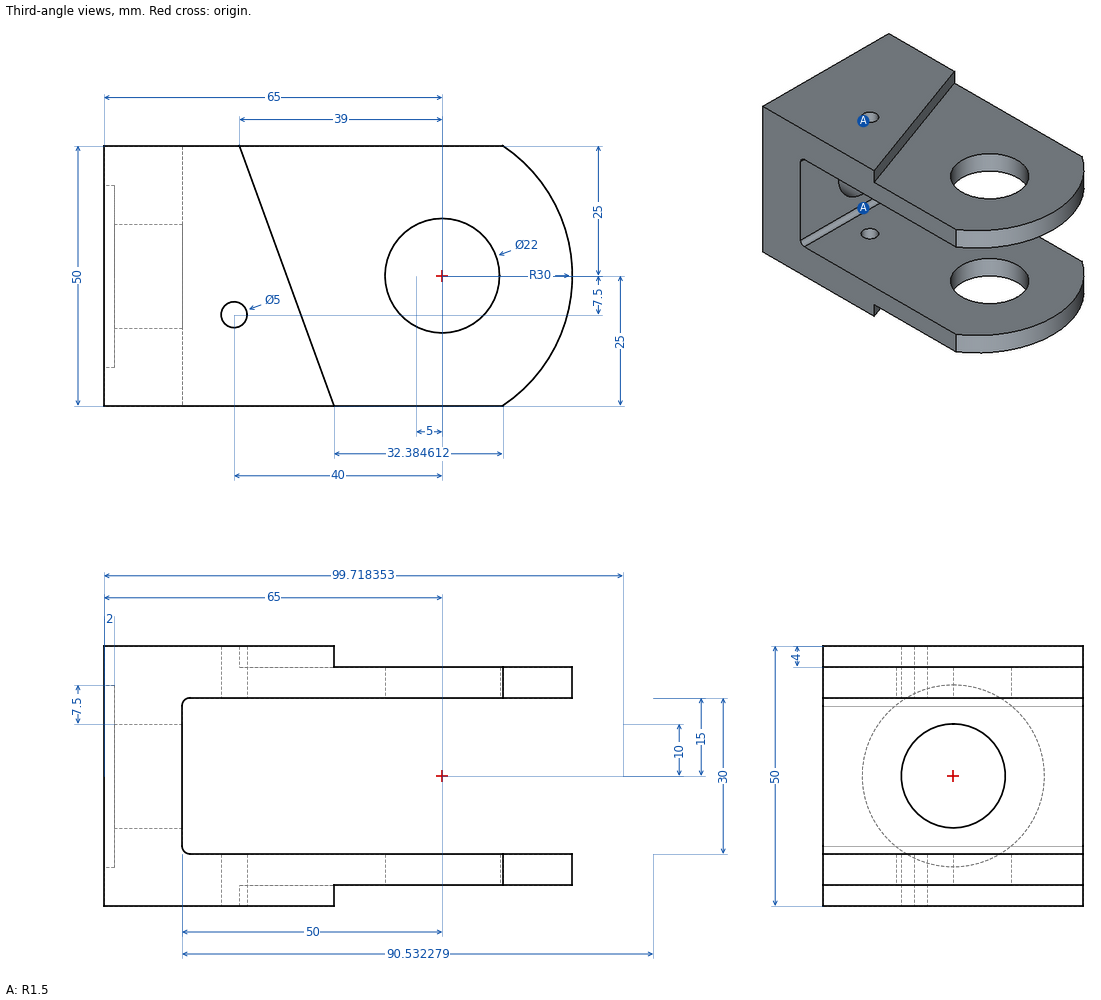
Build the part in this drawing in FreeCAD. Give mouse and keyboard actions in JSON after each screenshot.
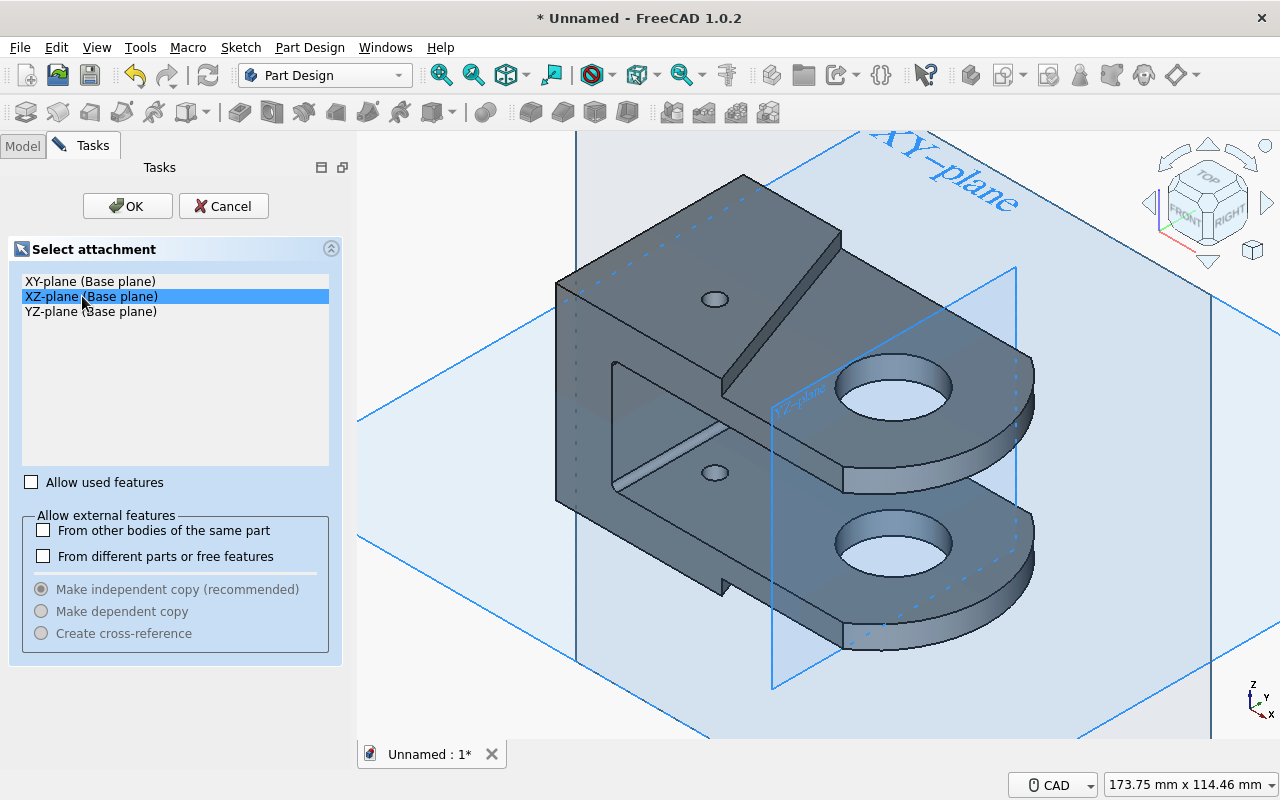
{"action": "left_click", "coordinate": [128, 206]}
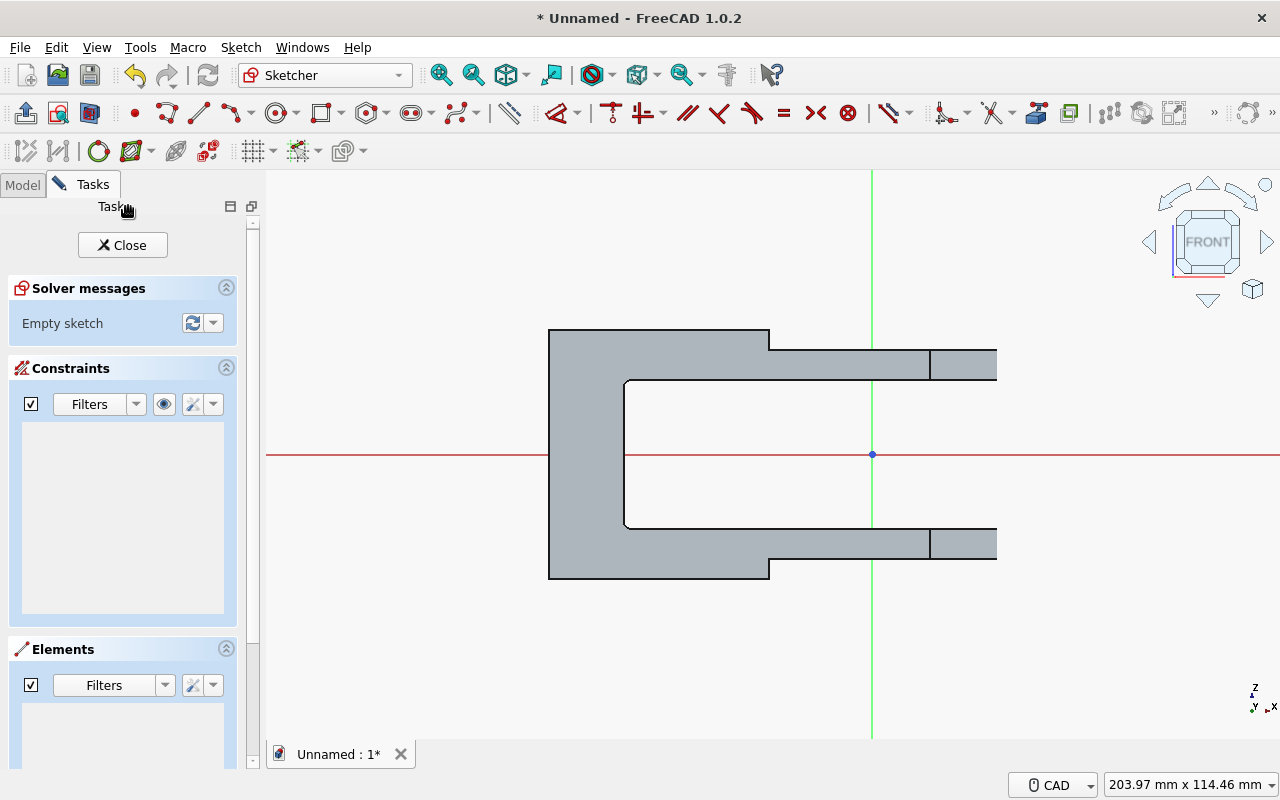
{"action": "left_click", "coordinate": [90, 114]}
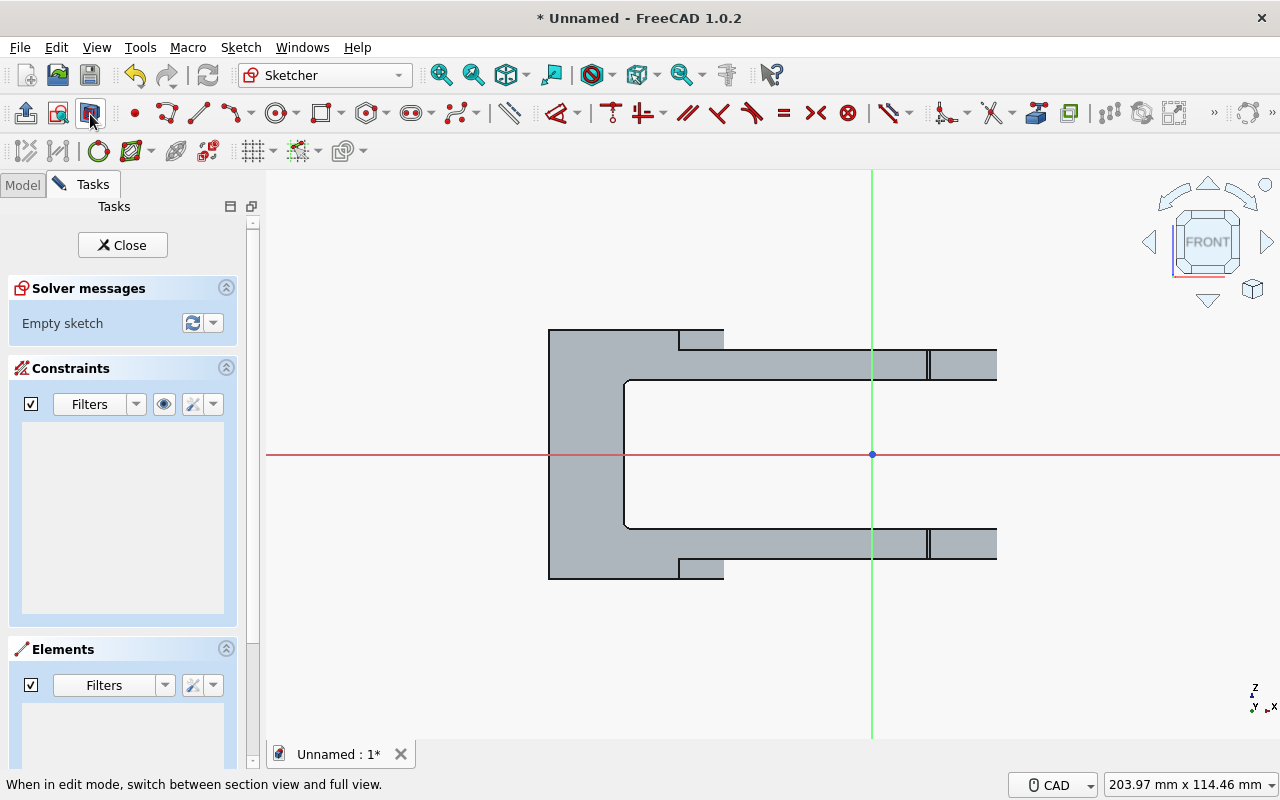
{"action": "left_click", "coordinate": [168, 114]}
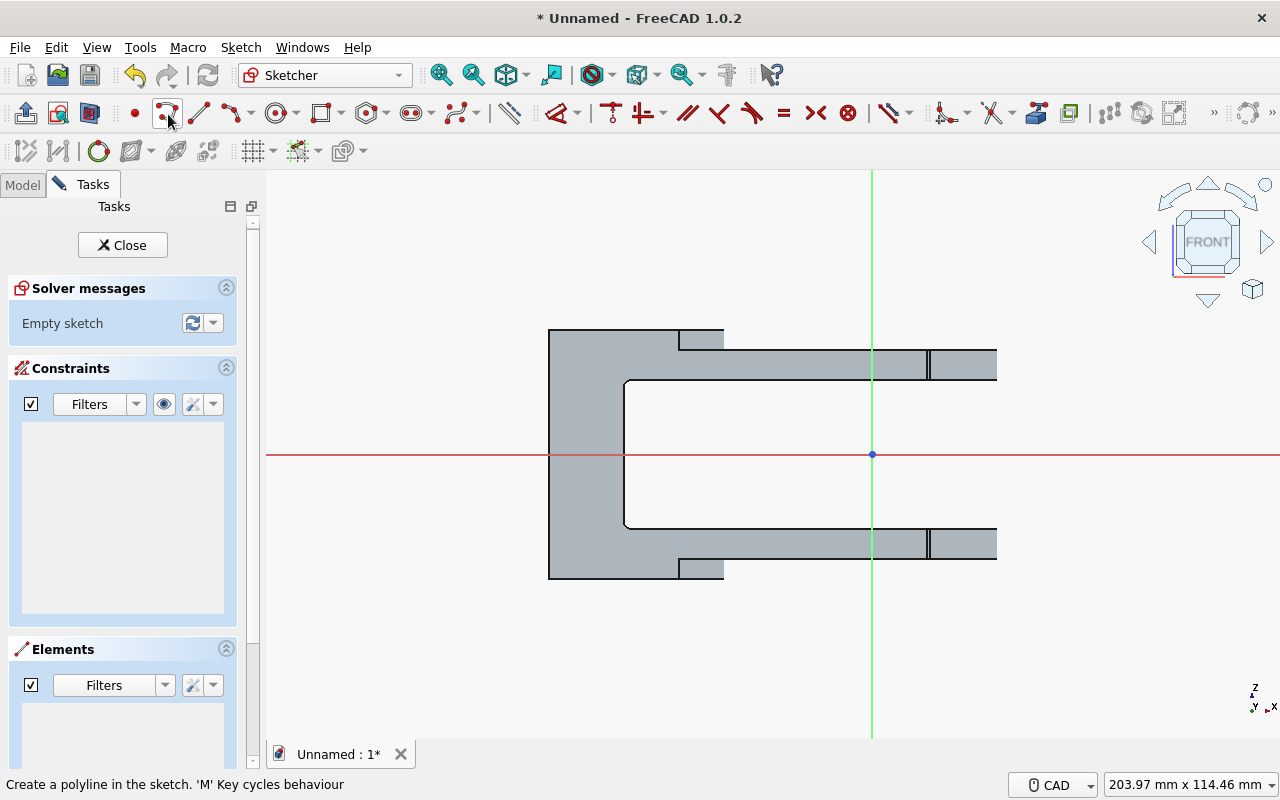
{"action": "left_click", "coordinate": [1045, 454]}
{"action": "left_click", "coordinate": [549, 446]}
{"action": "left_click", "coordinate": [549, 368]}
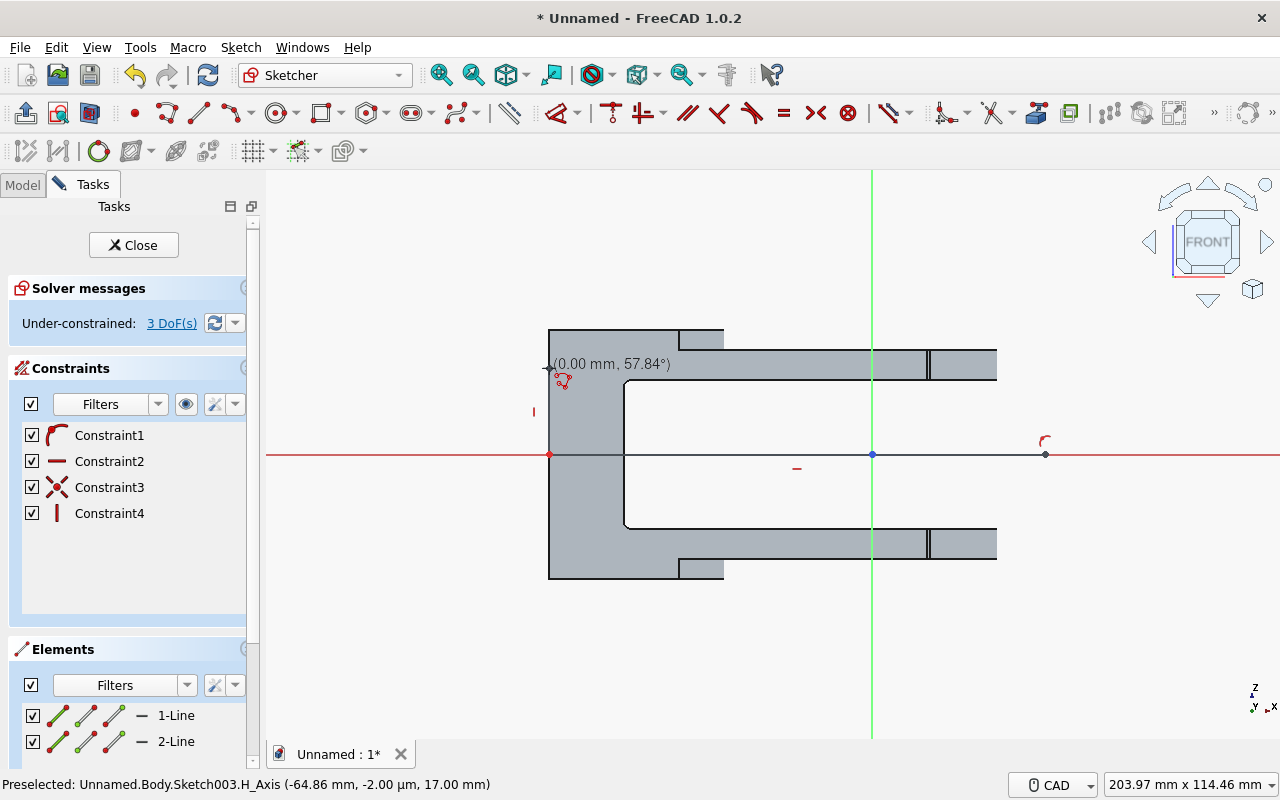
{"action": "scroll", "coordinate": [559, 368], "scroll_direction": "up", "scroll_amount": 3}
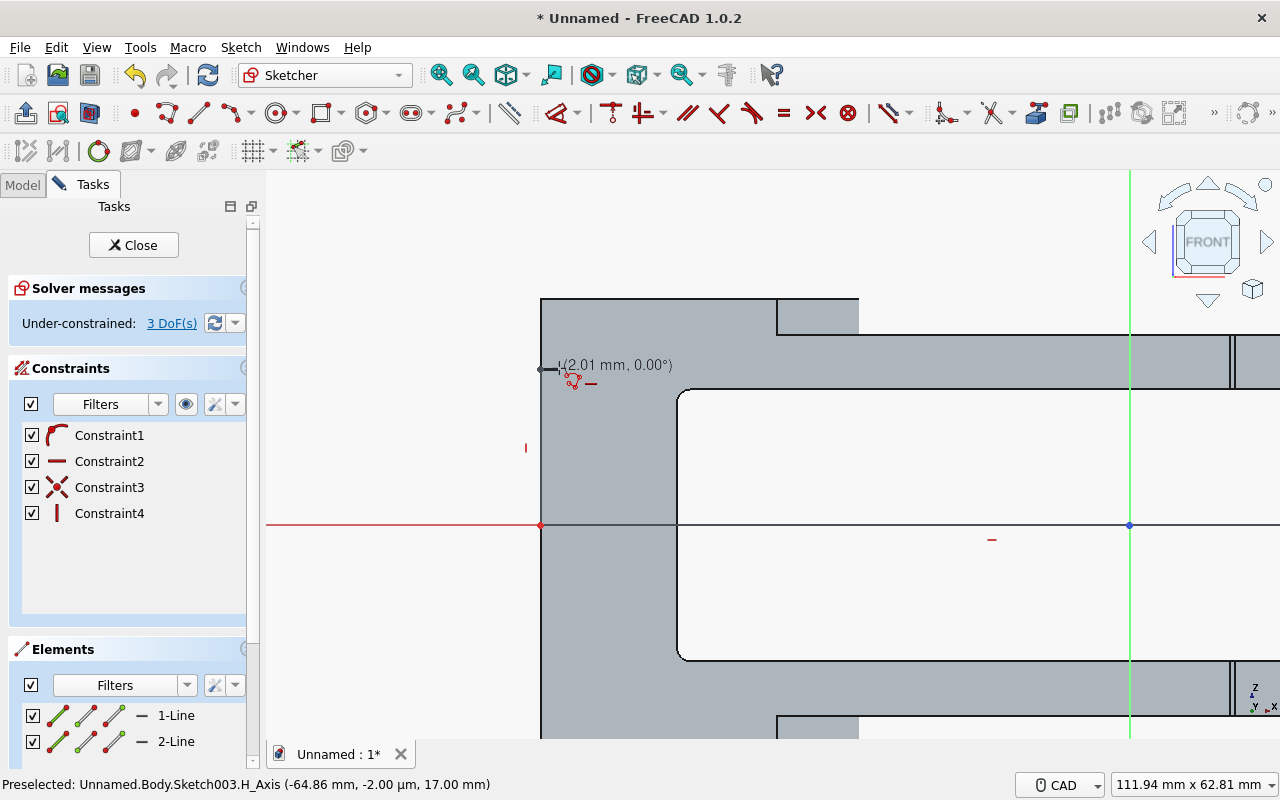
{"action": "left_click", "coordinate": [559, 368]}
{"action": "left_click", "coordinate": [559, 435]}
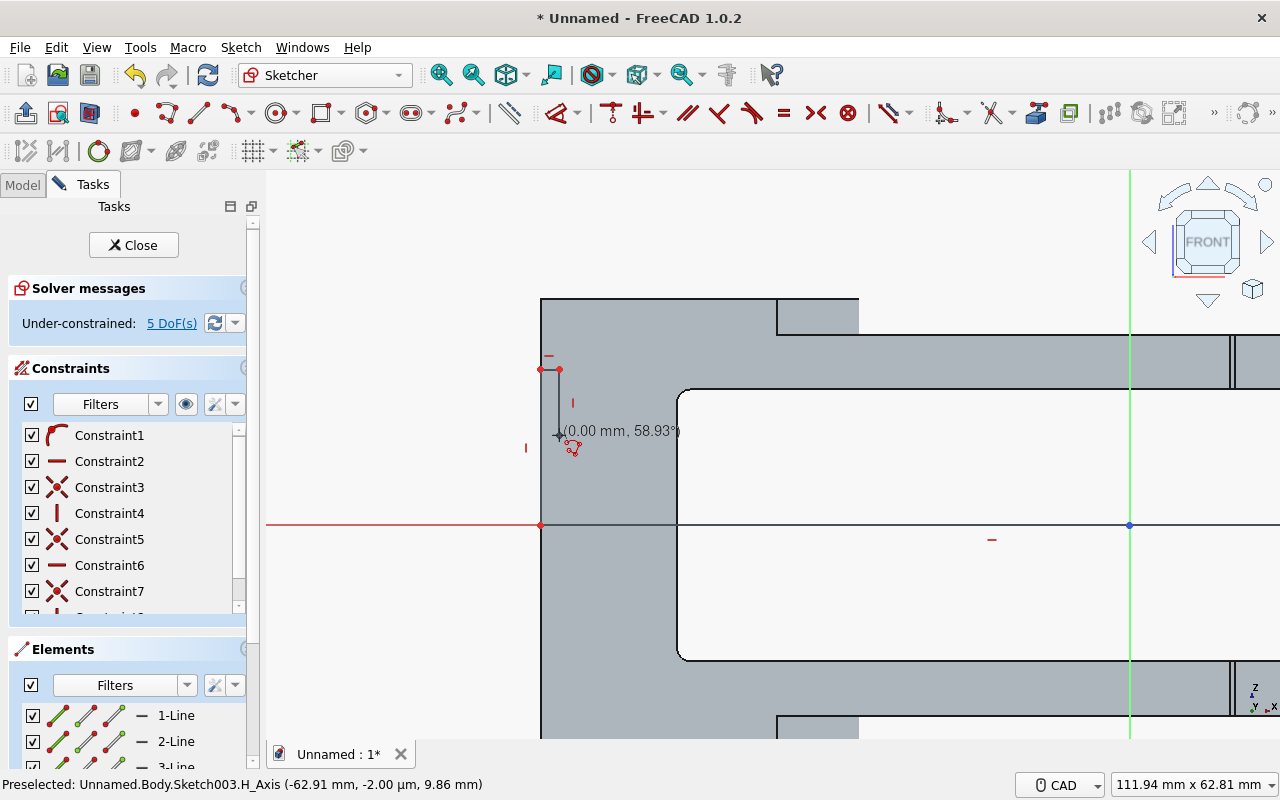
{"action": "scroll", "coordinate": [294, 472], "scroll_direction": "down", "scroll_amount": 2}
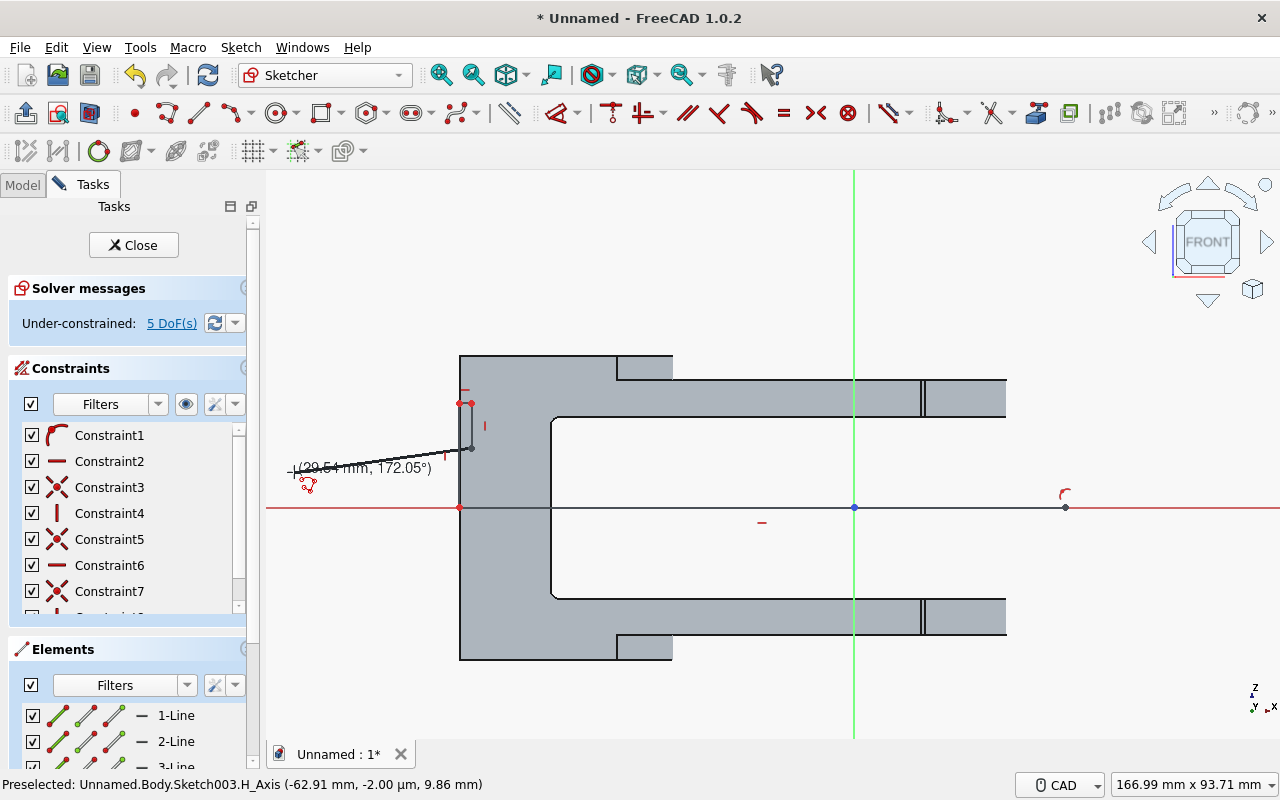
{"action": "left_click", "coordinate": [1065, 447]}
{"action": "left_click", "coordinate": [1065, 508]}
{"action": "key", "text": "Escape"}
{"action": "key", "text": "Escape"}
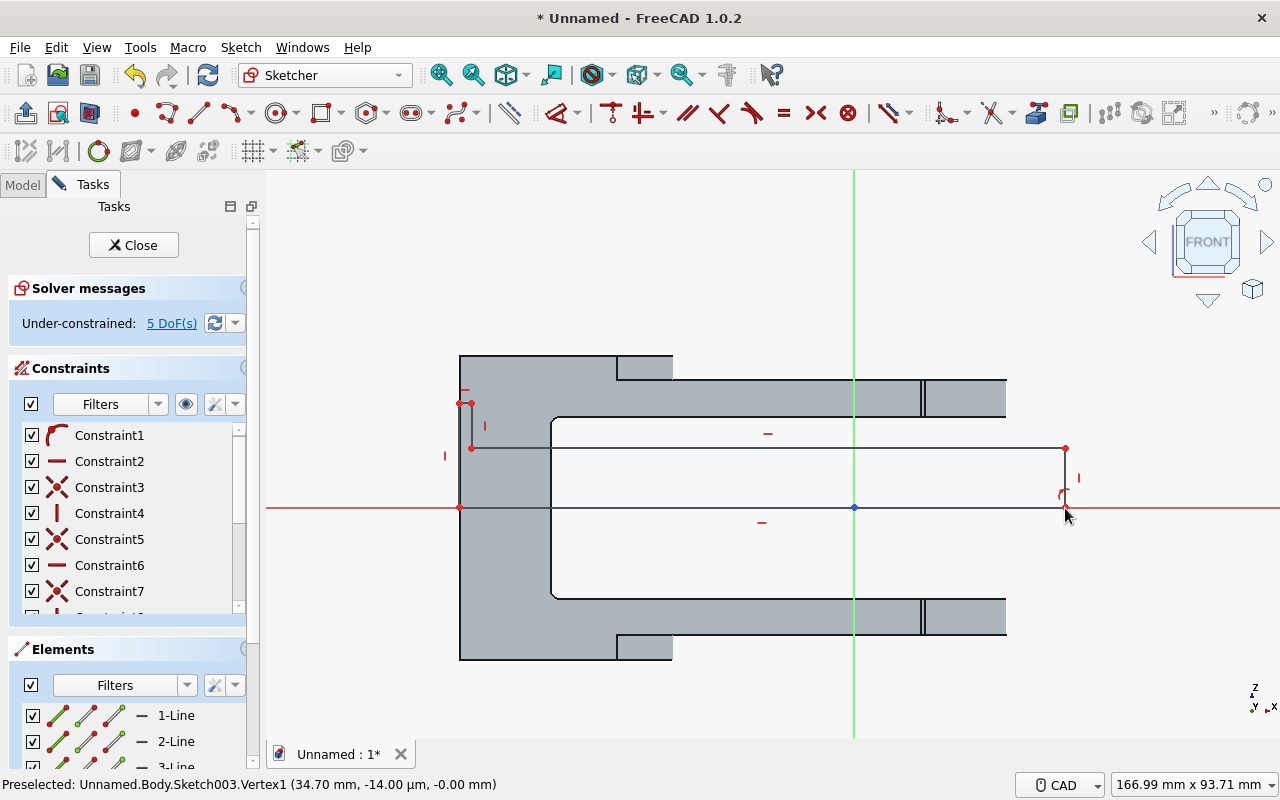
{"action": "left_click", "coordinate": [556, 114]}